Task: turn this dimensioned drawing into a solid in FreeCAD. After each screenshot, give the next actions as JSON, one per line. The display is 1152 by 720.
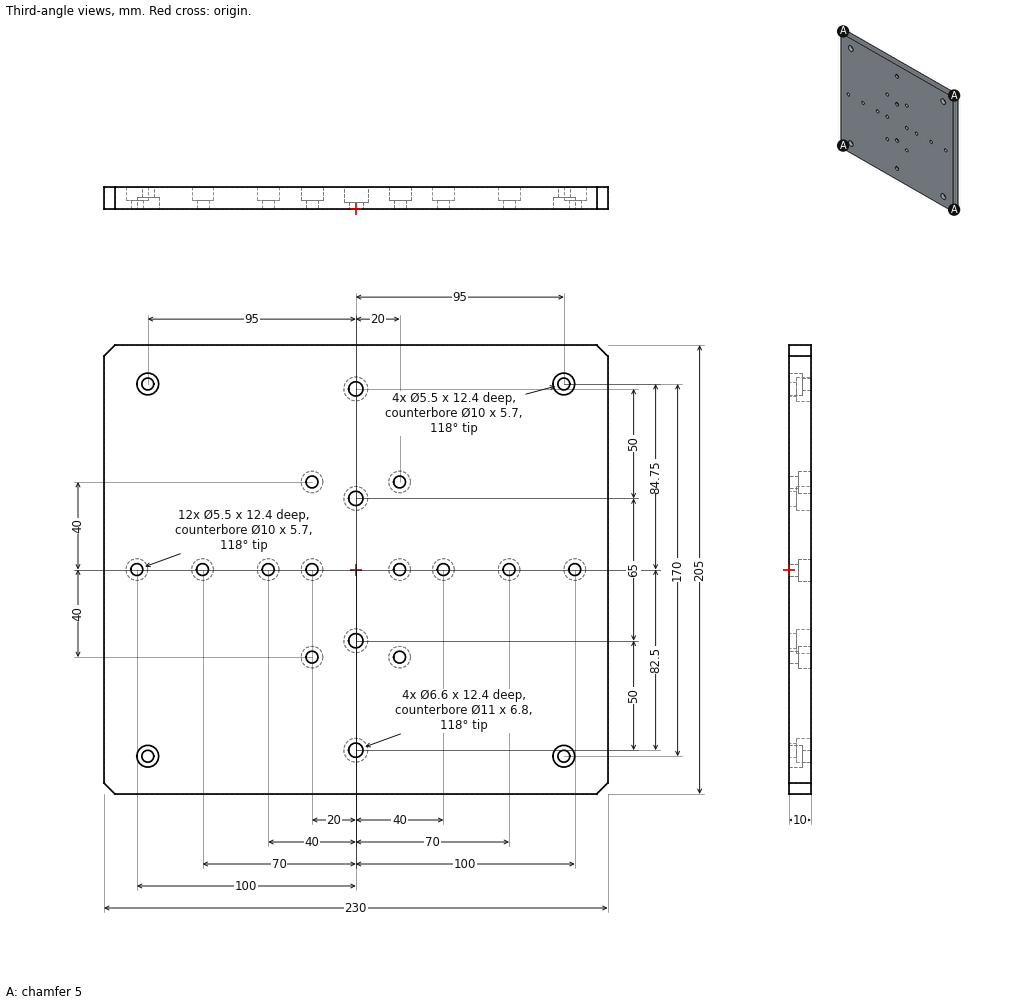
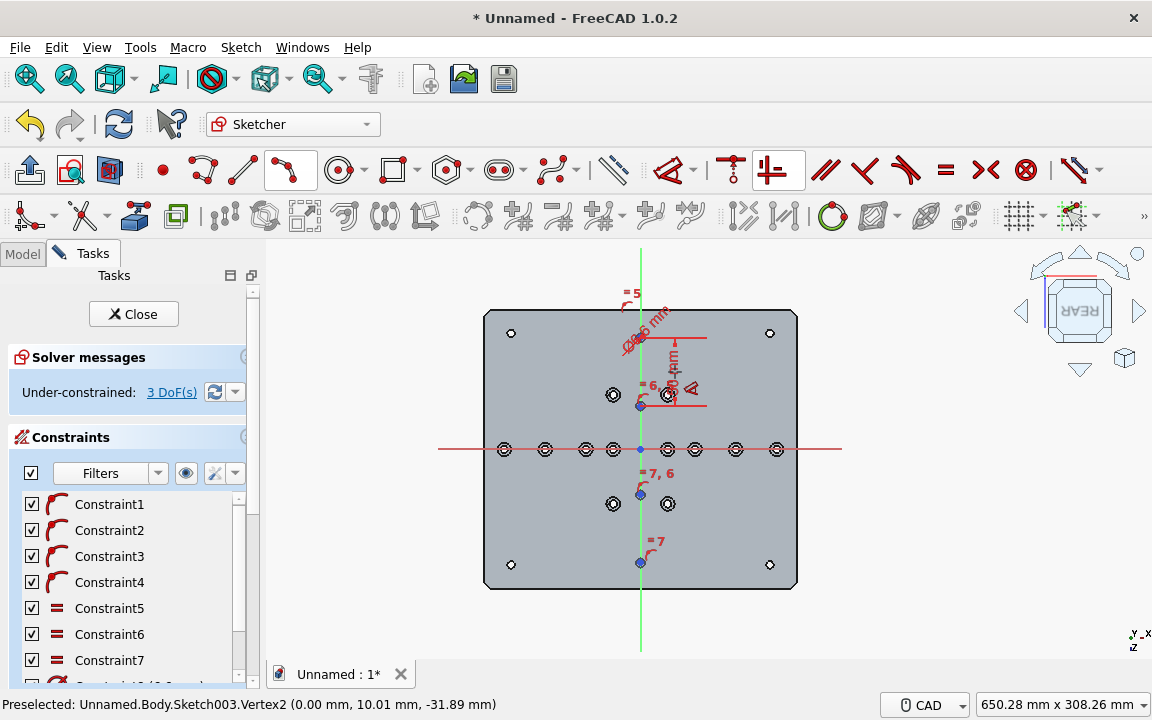
{"action": "left_click", "coordinate": [641, 406]}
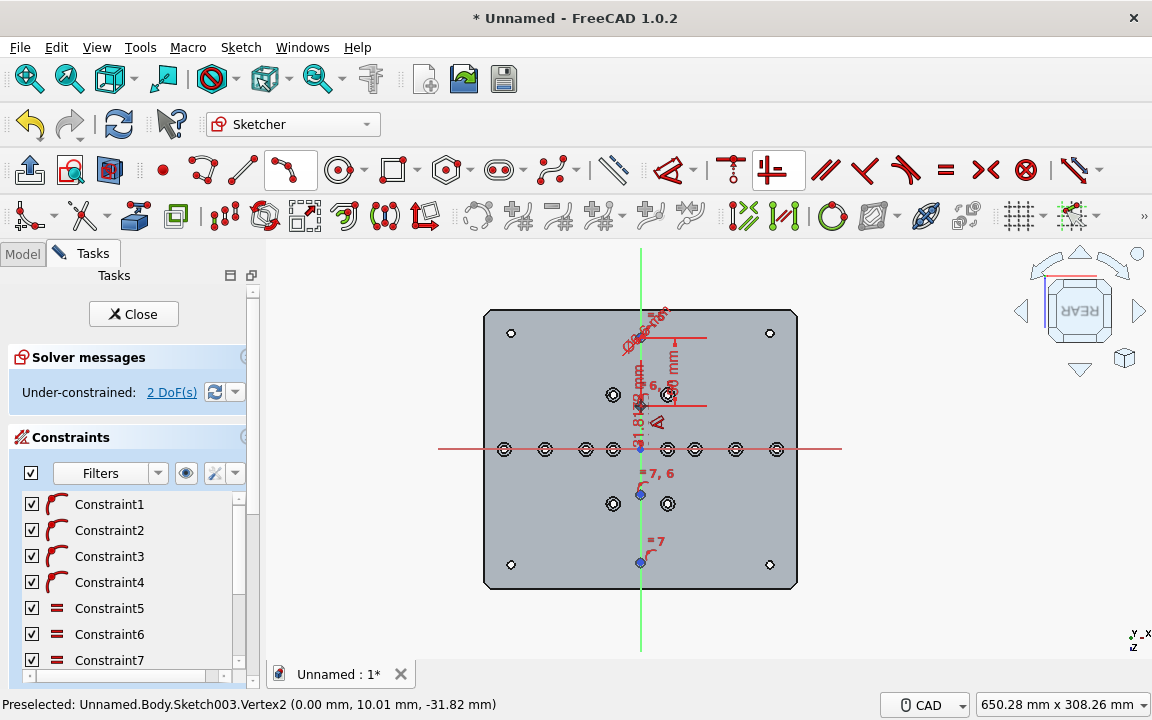
{"action": "left_click", "coordinate": [641, 495]}
{"action": "left_click", "coordinate": [675, 430]}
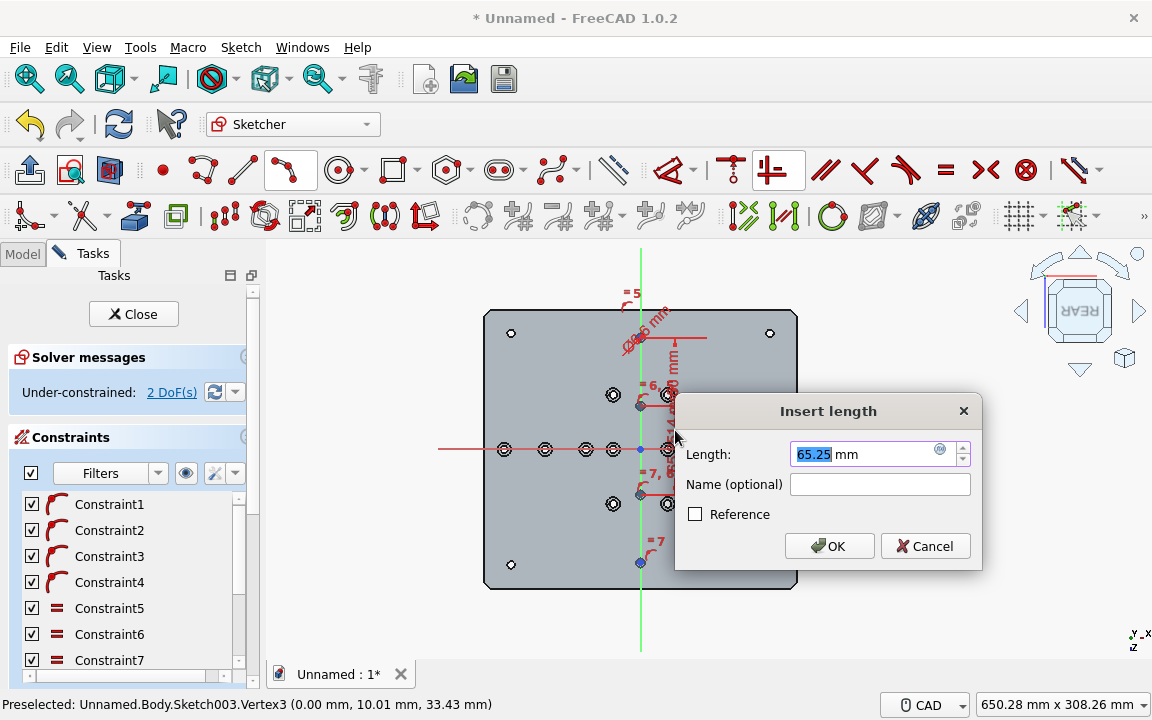
{"action": "type", "text": "65"}
{"action": "key", "text": "Return"}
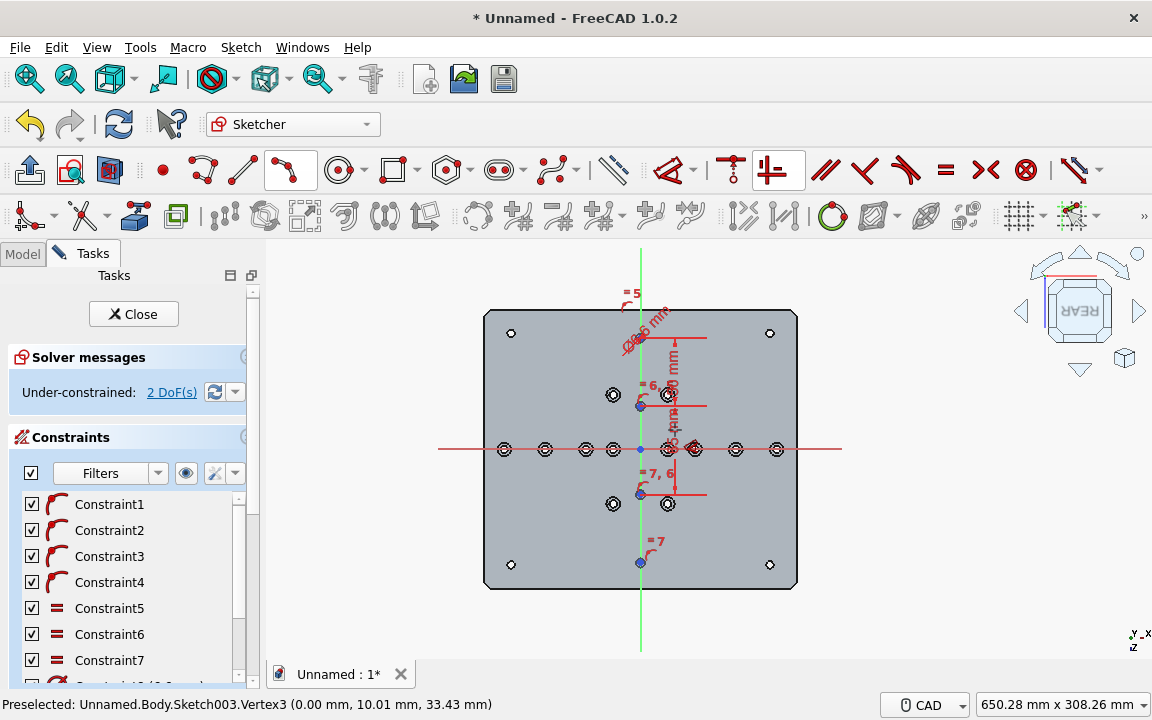
{"action": "left_click", "coordinate": [641, 495]}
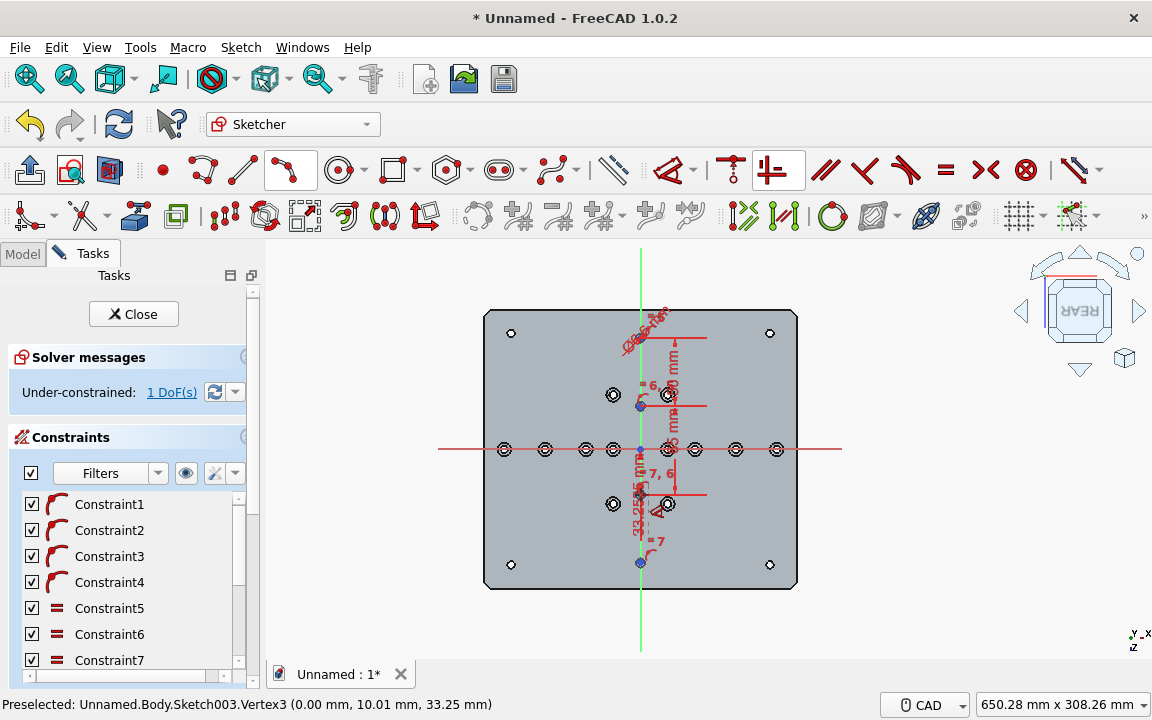
{"action": "left_click", "coordinate": [641, 563]}
{"action": "left_click", "coordinate": [675, 529]}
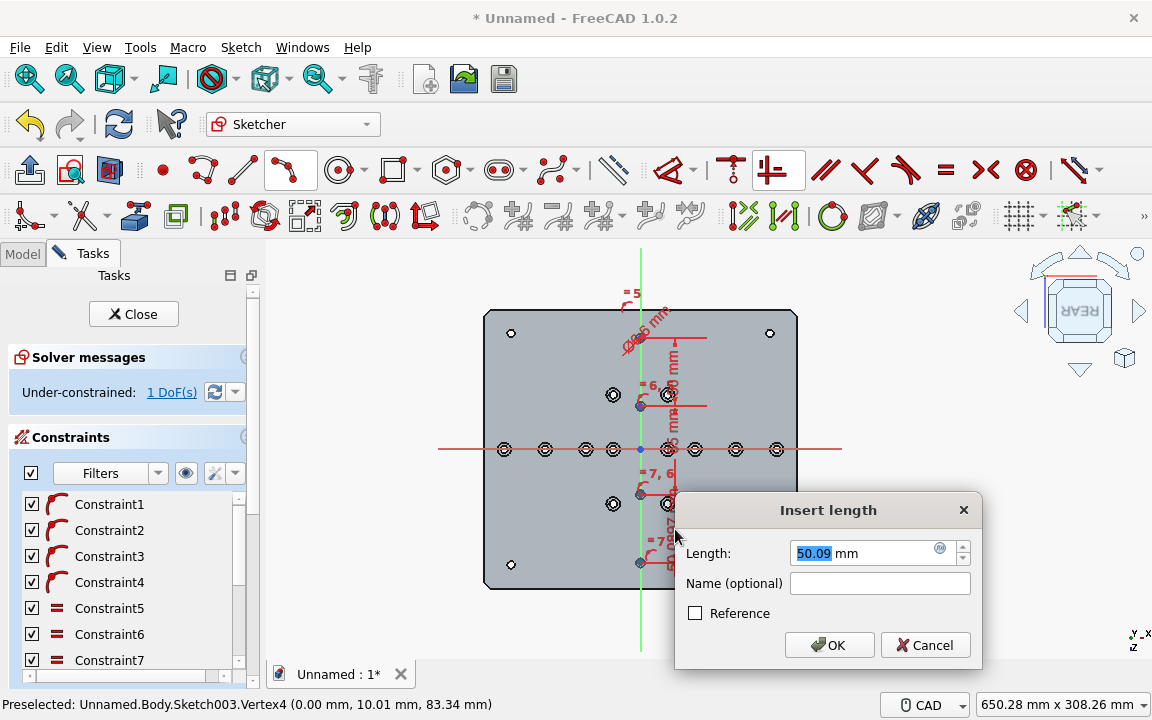
{"action": "type", "text": "50"}
{"action": "key", "text": "Return"}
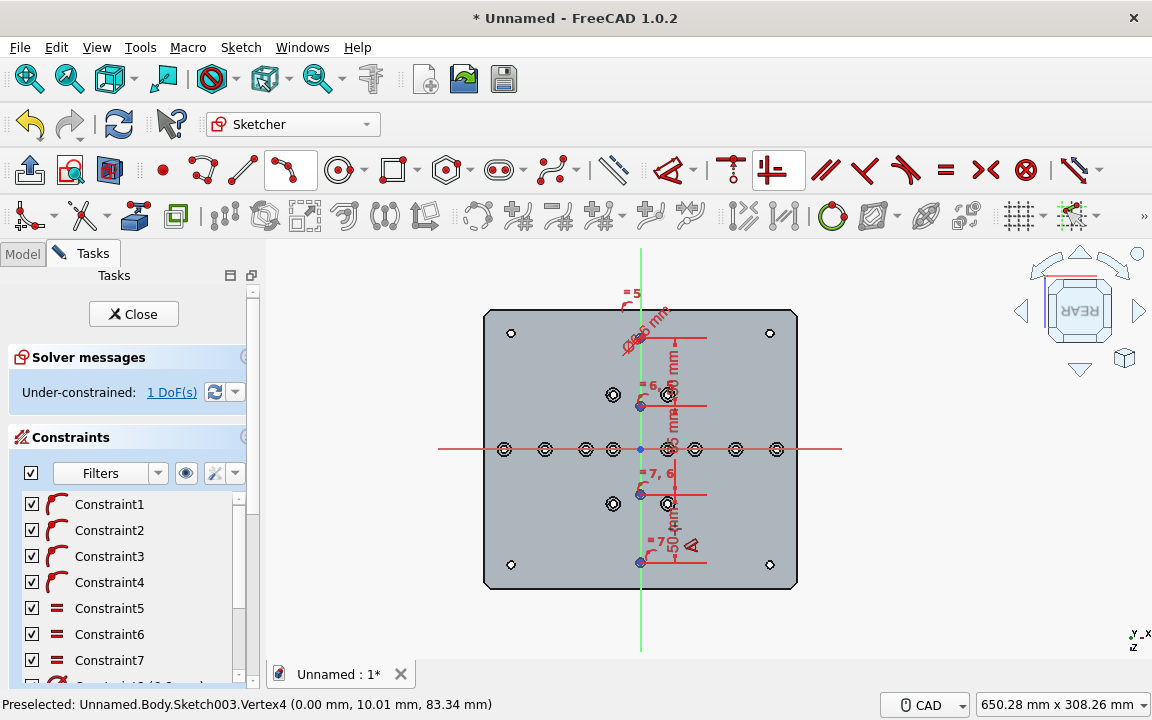
{"action": "left_click", "coordinate": [641, 338]}
{"action": "left_click", "coordinate": [675, 394]}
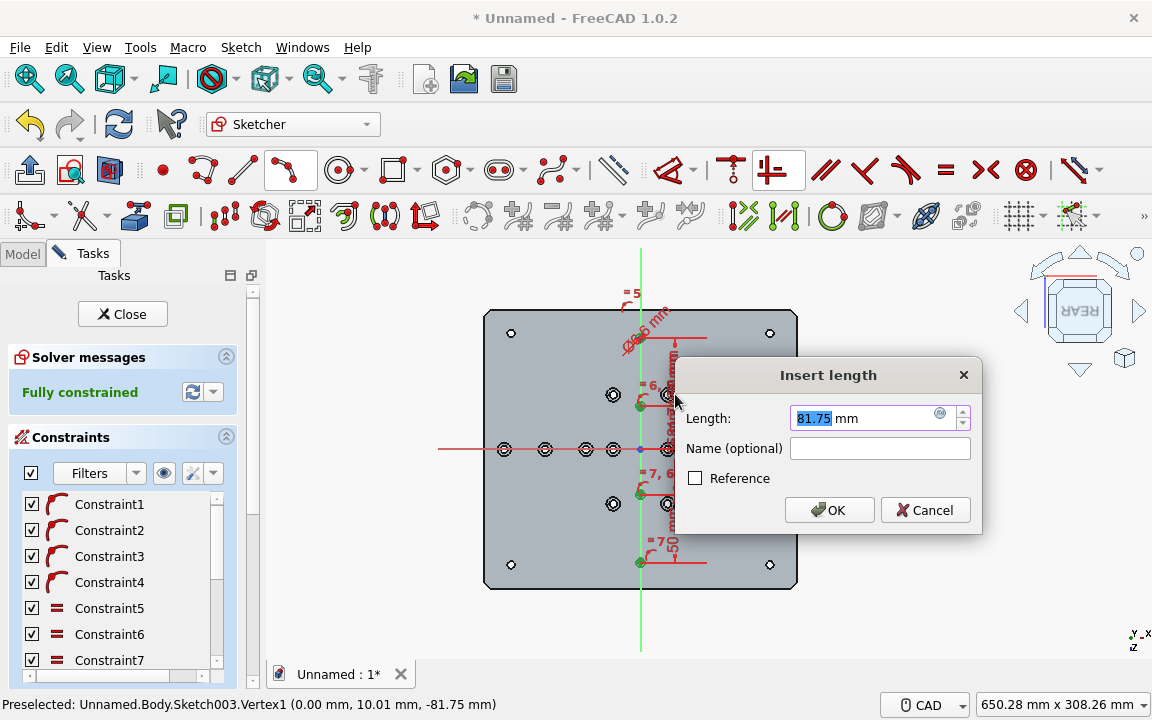
{"action": "type", "text": "82.5"}
{"action": "key", "text": "Return"}
{"action": "key", "text": "Escape"}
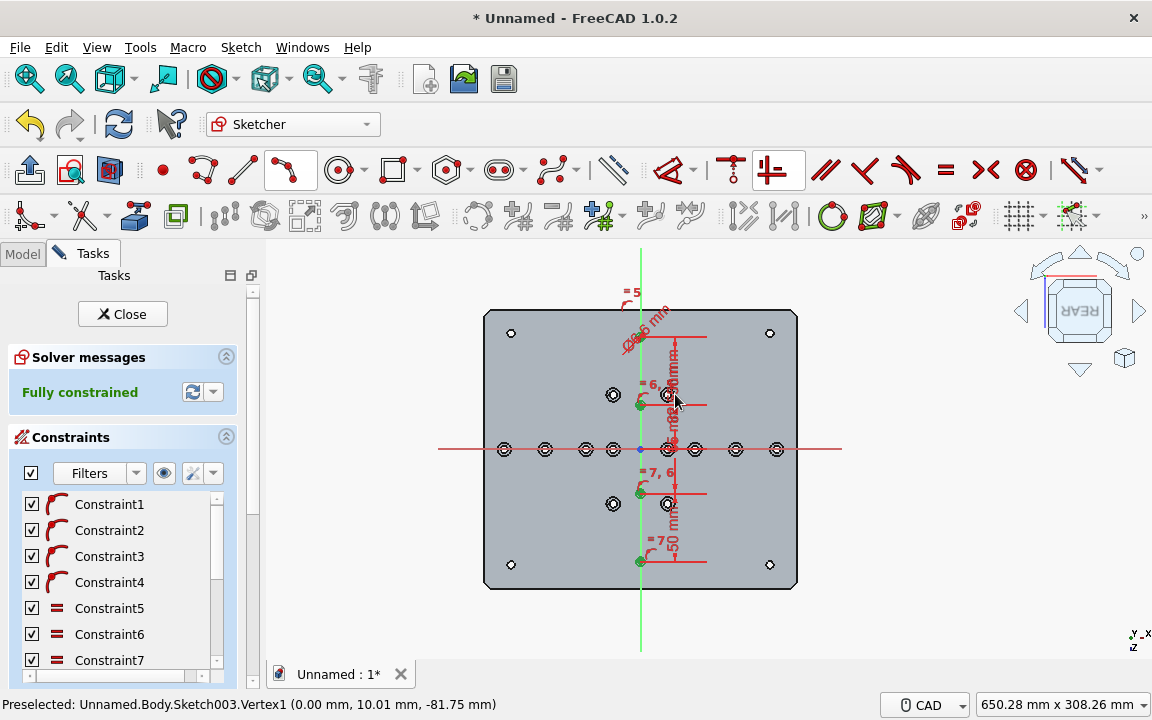
{"action": "left_click", "coordinate": [123, 314]}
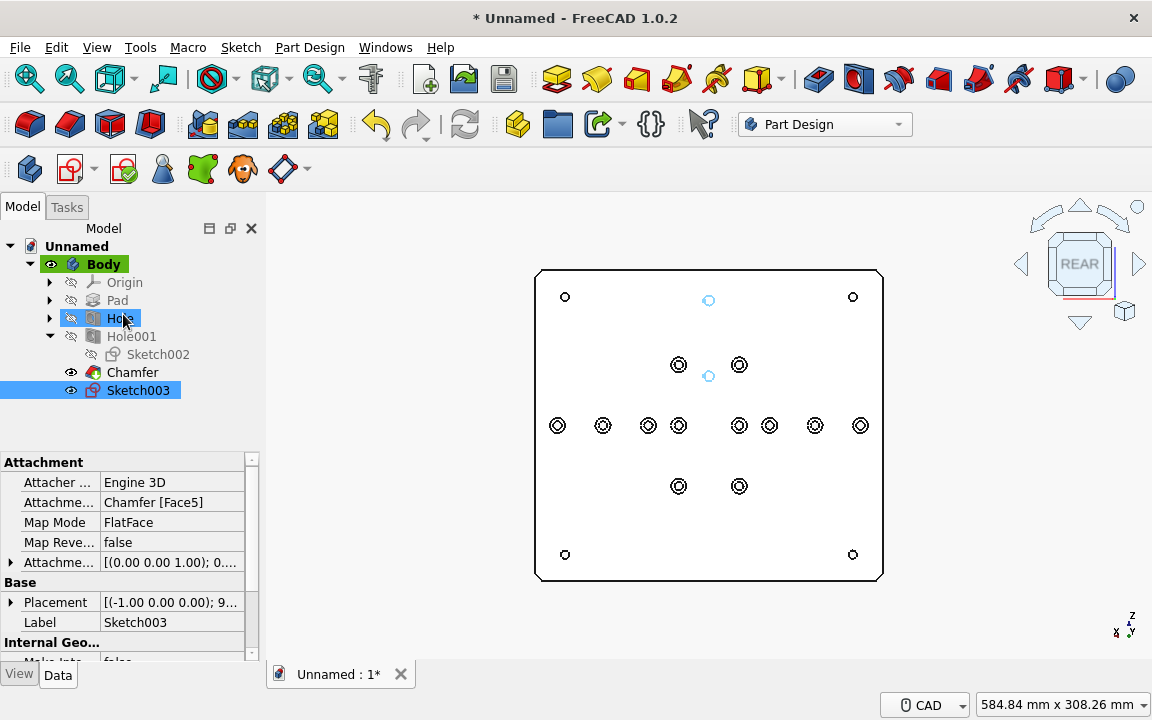
{"action": "left_click", "coordinate": [860, 80]}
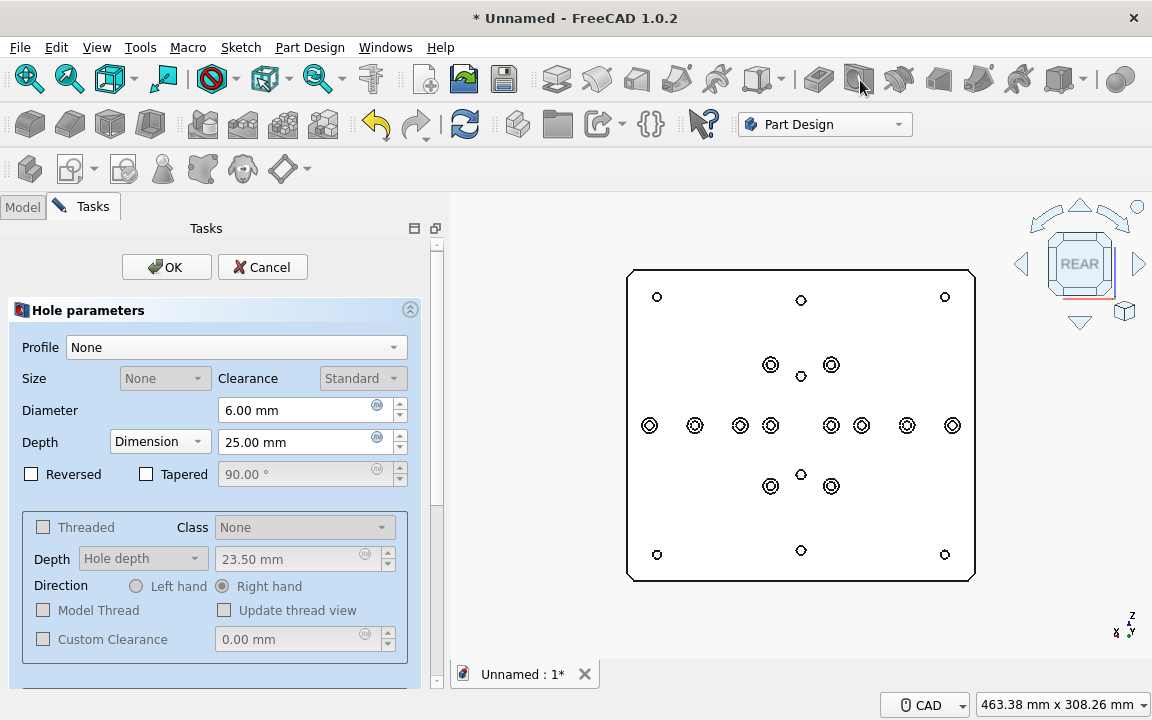
{"action": "triple_click", "coordinate": [305, 410]}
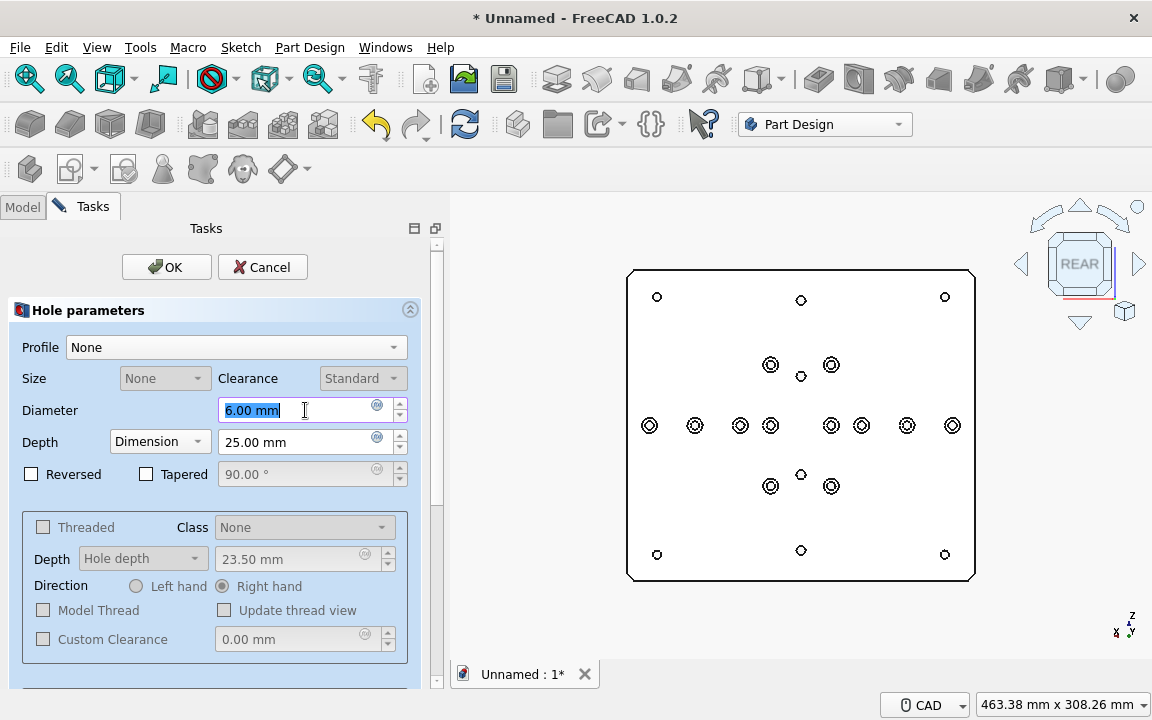
{"action": "type", "text": "6.6"}
{"action": "key", "text": "Tab"}